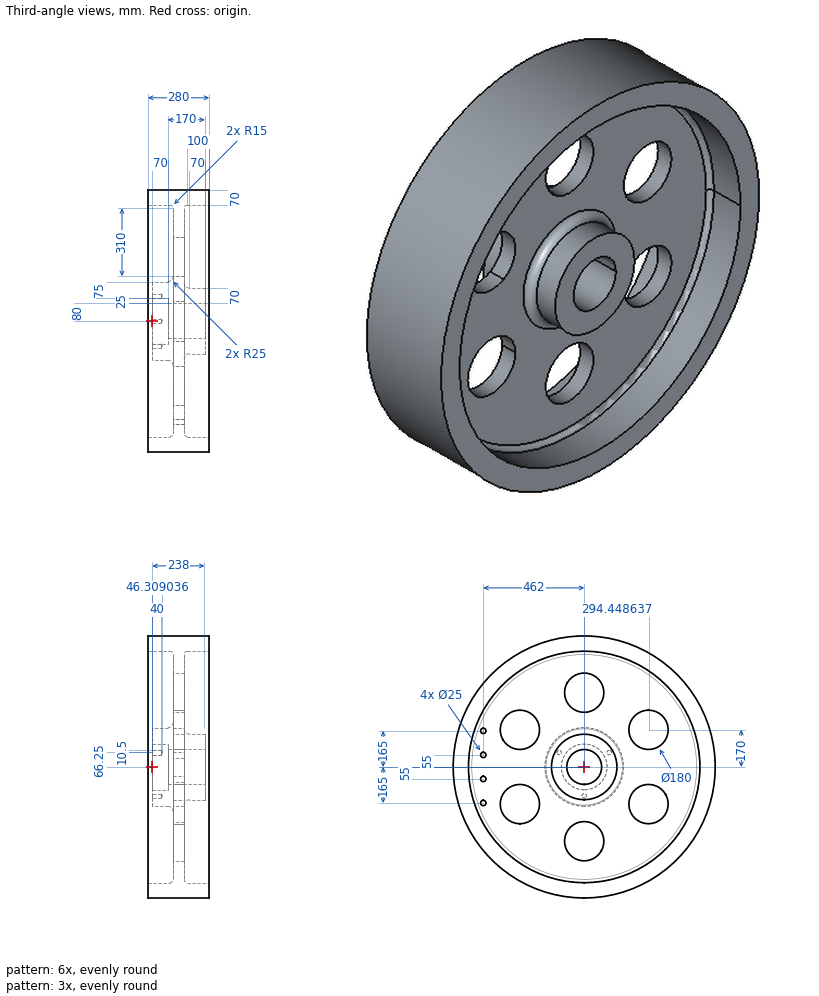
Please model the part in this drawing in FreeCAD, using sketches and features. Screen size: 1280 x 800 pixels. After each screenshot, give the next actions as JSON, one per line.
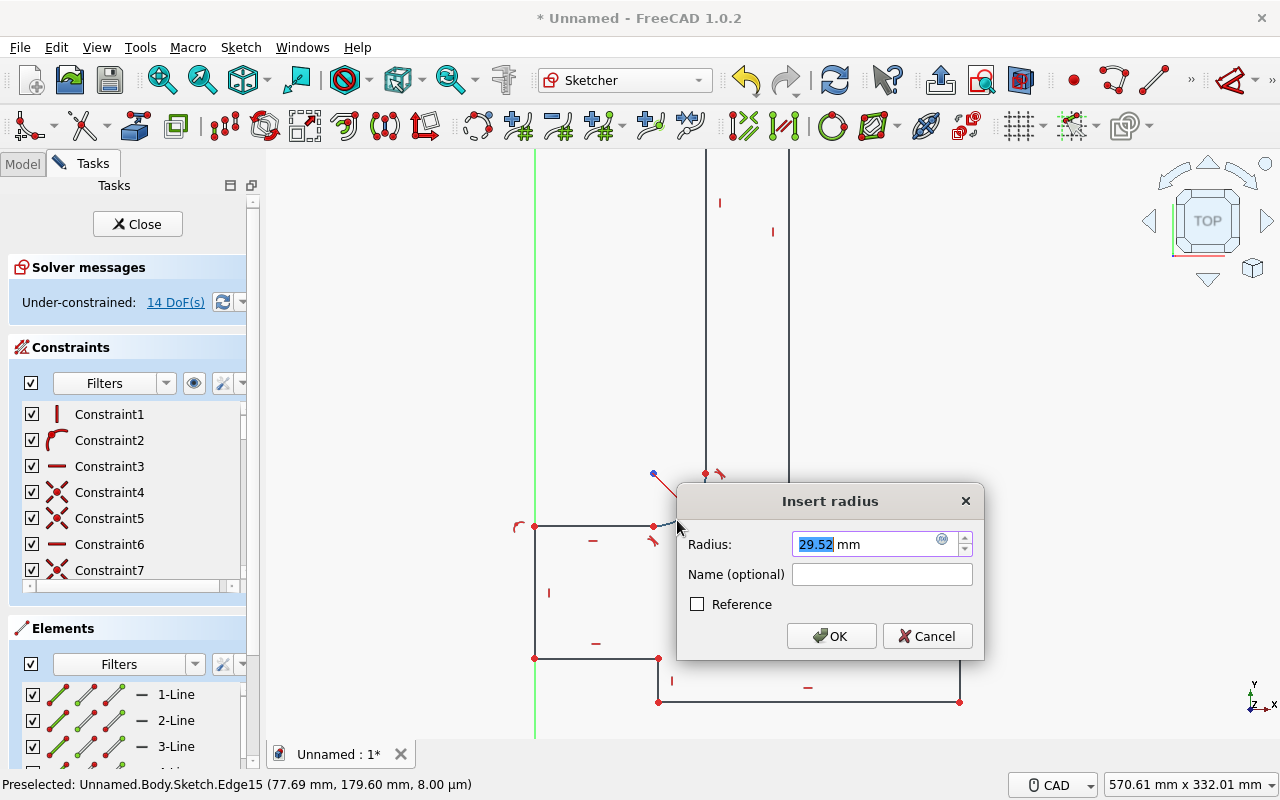
{"action": "type", "text": "25"}
{"action": "key", "text": "Return"}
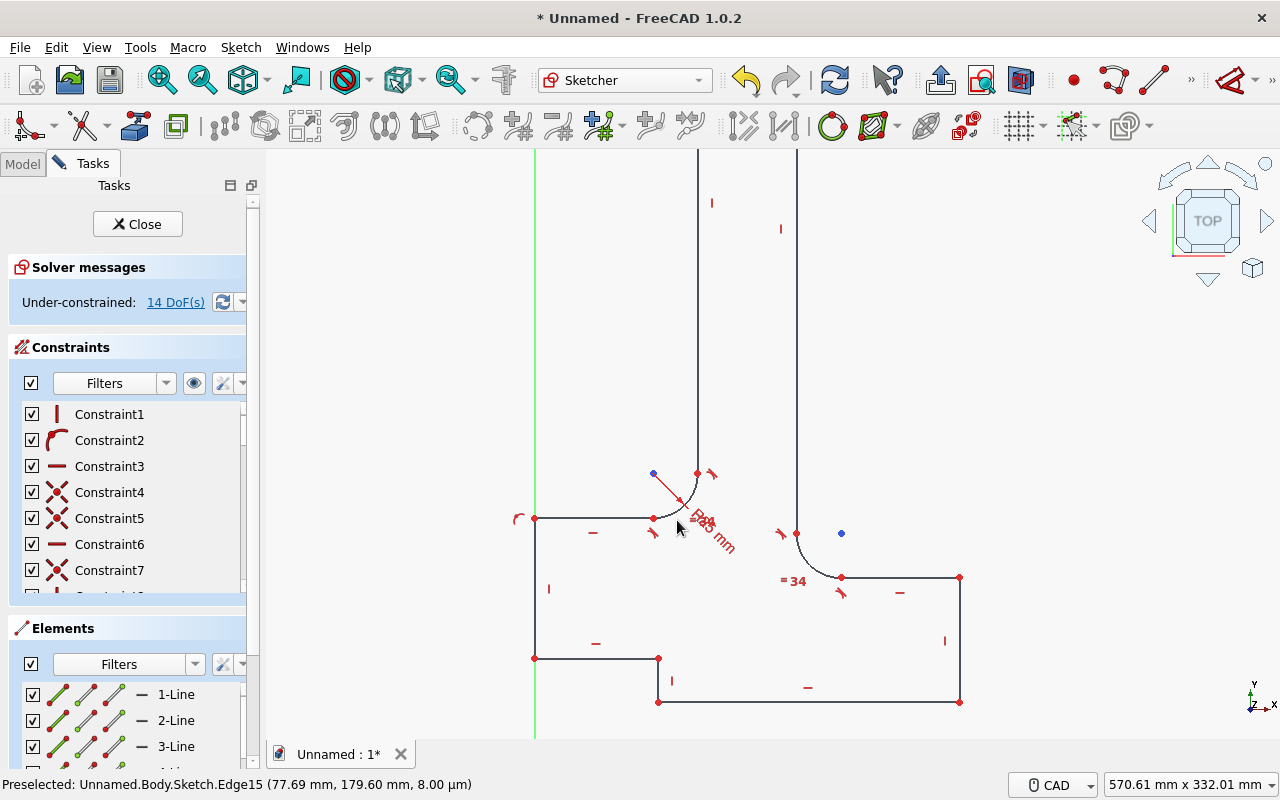
{"action": "scroll", "coordinate": [679, 523], "scroll_direction": "down", "scroll_amount": 5}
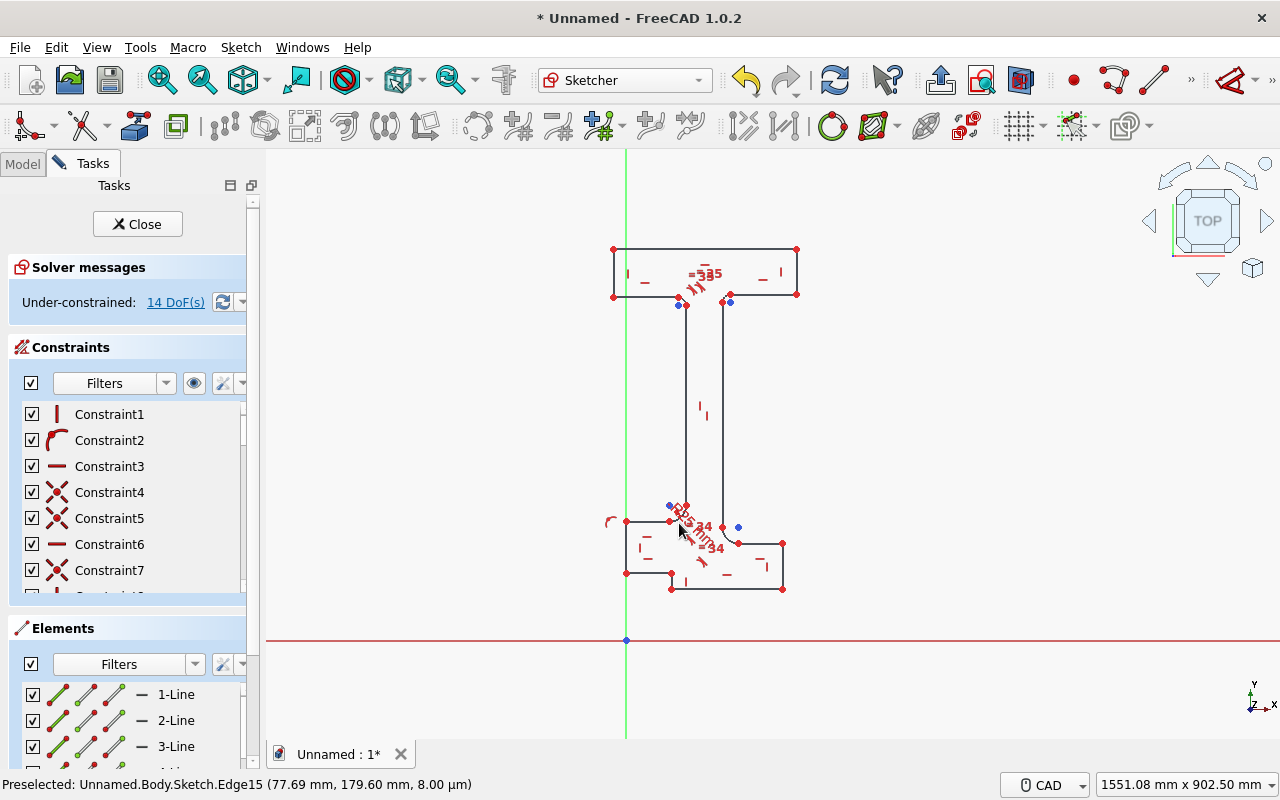
{"action": "scroll", "coordinate": [727, 296], "scroll_direction": "up", "scroll_amount": 7}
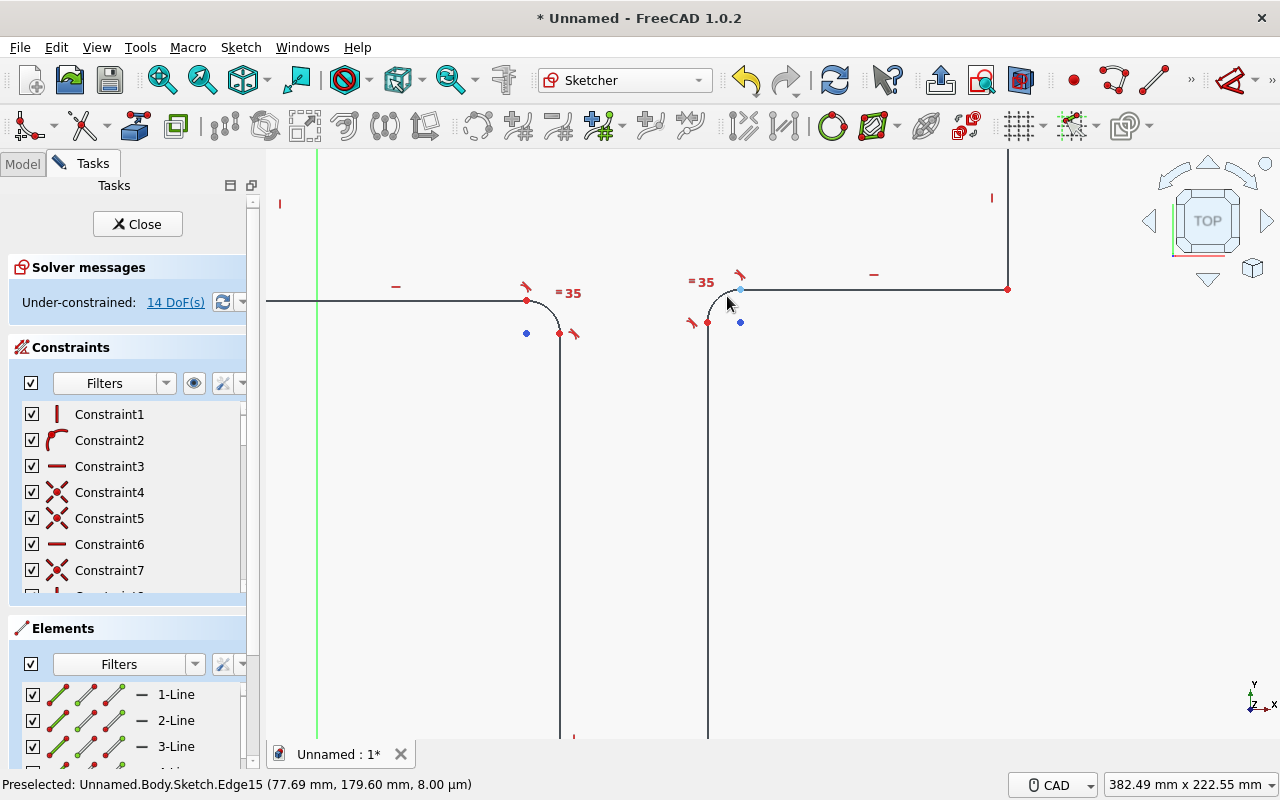
{"action": "left_click", "coordinate": [726, 293]}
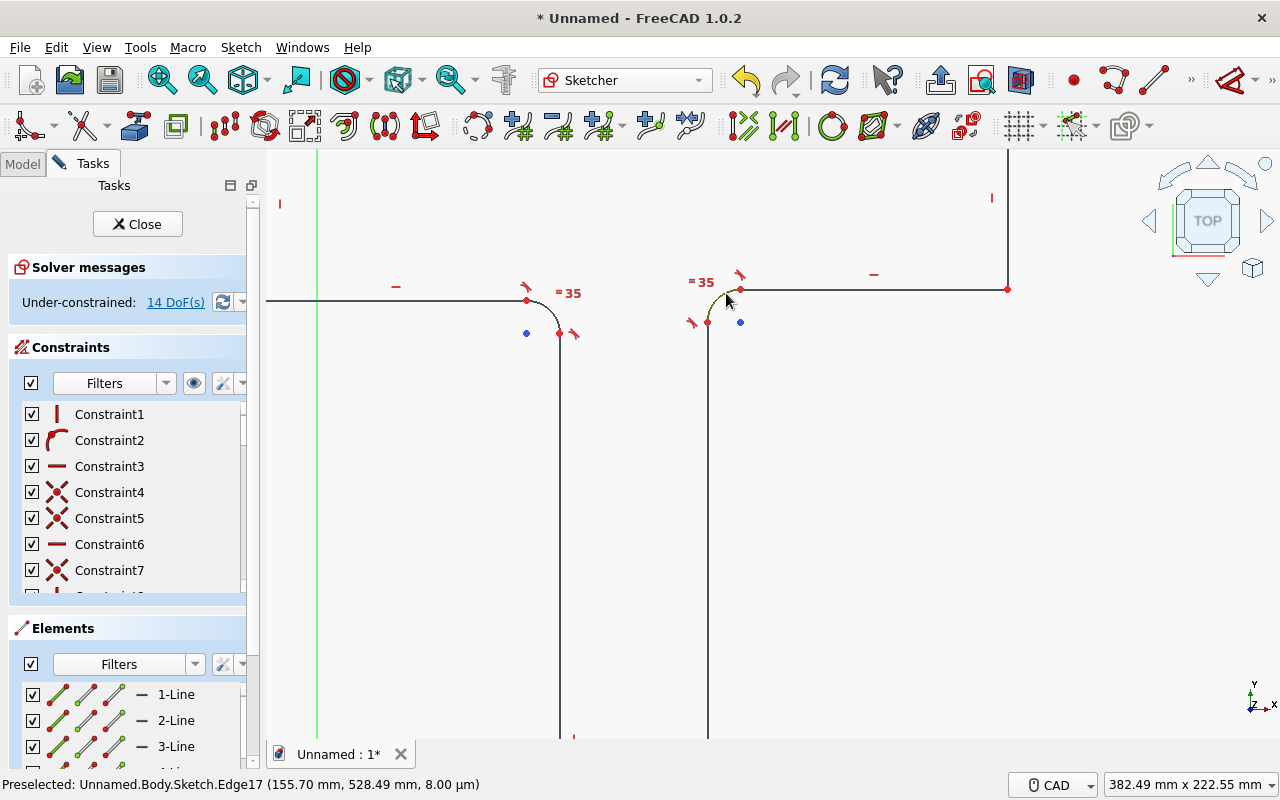
{"action": "left_click", "coordinate": [1258, 80]}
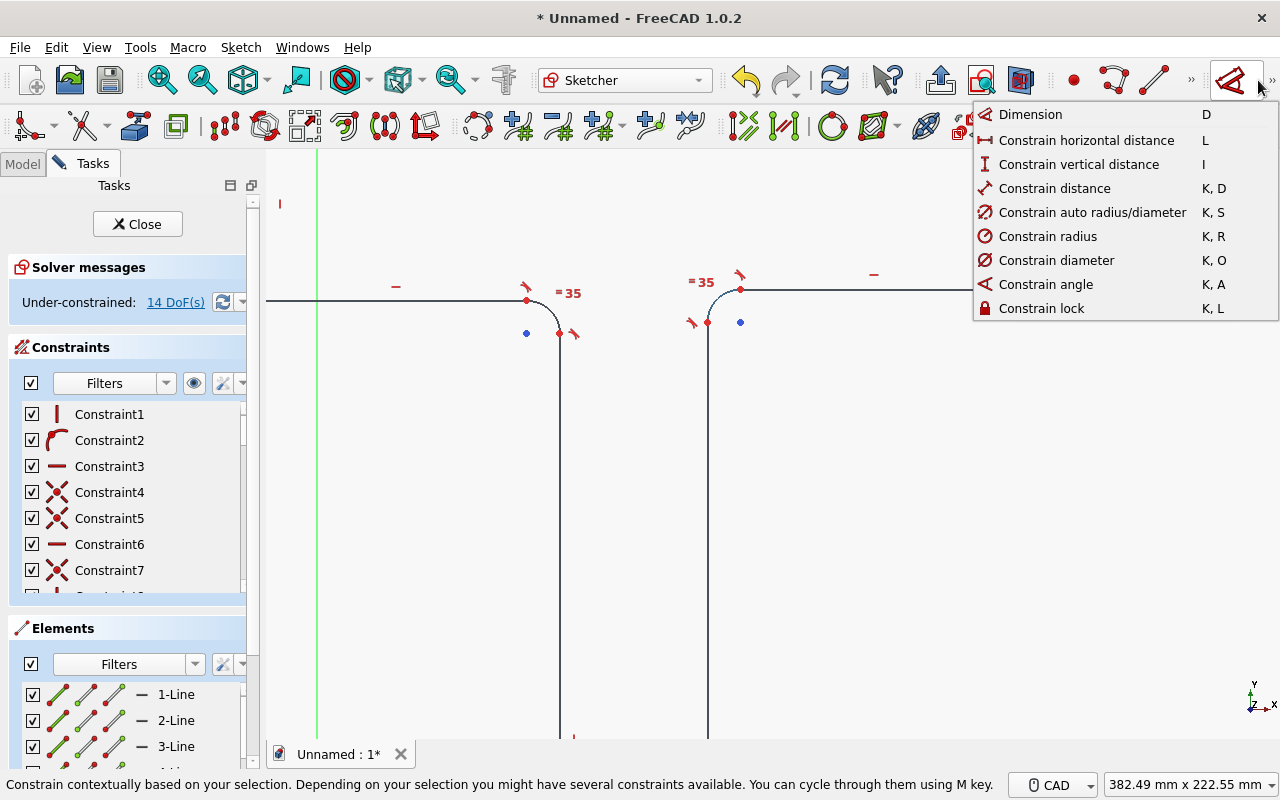
{"action": "left_click", "coordinate": [1126, 236]}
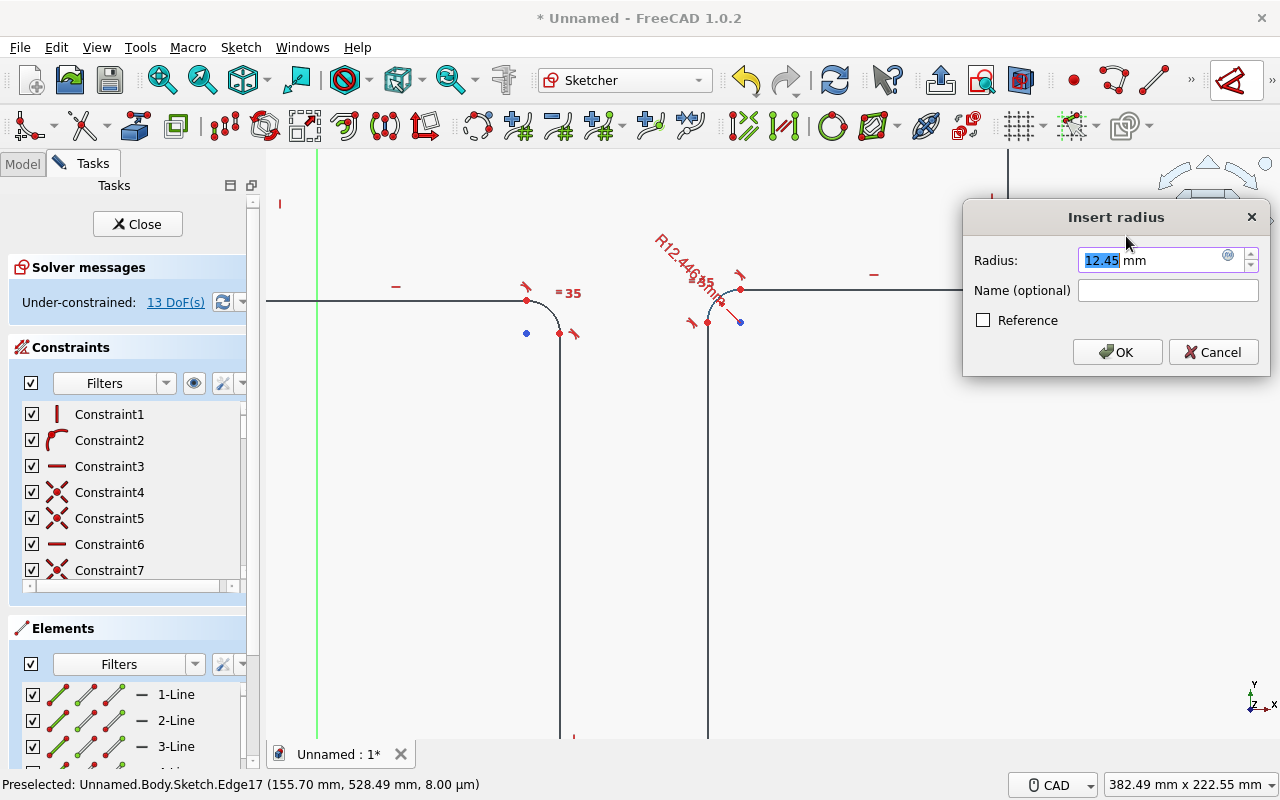
{"action": "type", "text": "15"}
{"action": "key", "text": "Return"}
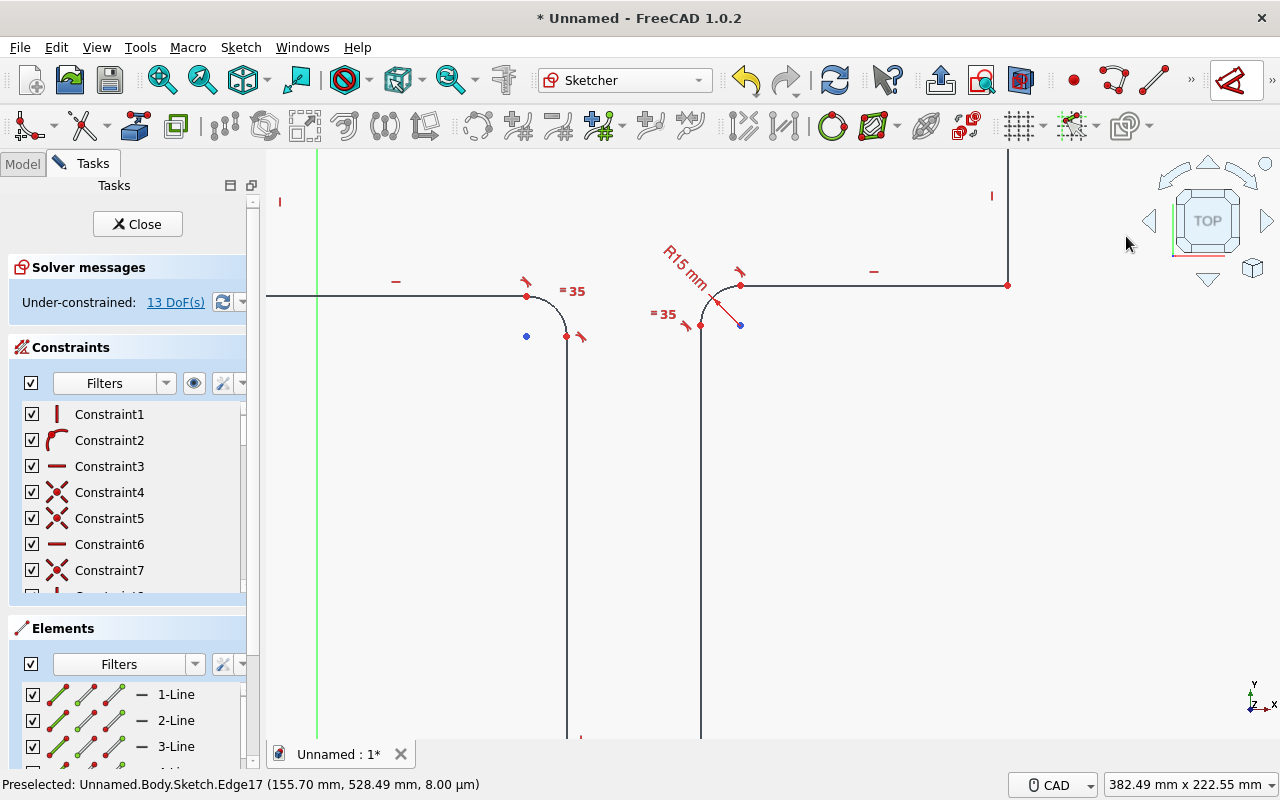
{"action": "scroll", "coordinate": [727, 296], "scroll_direction": "down", "scroll_amount": 7}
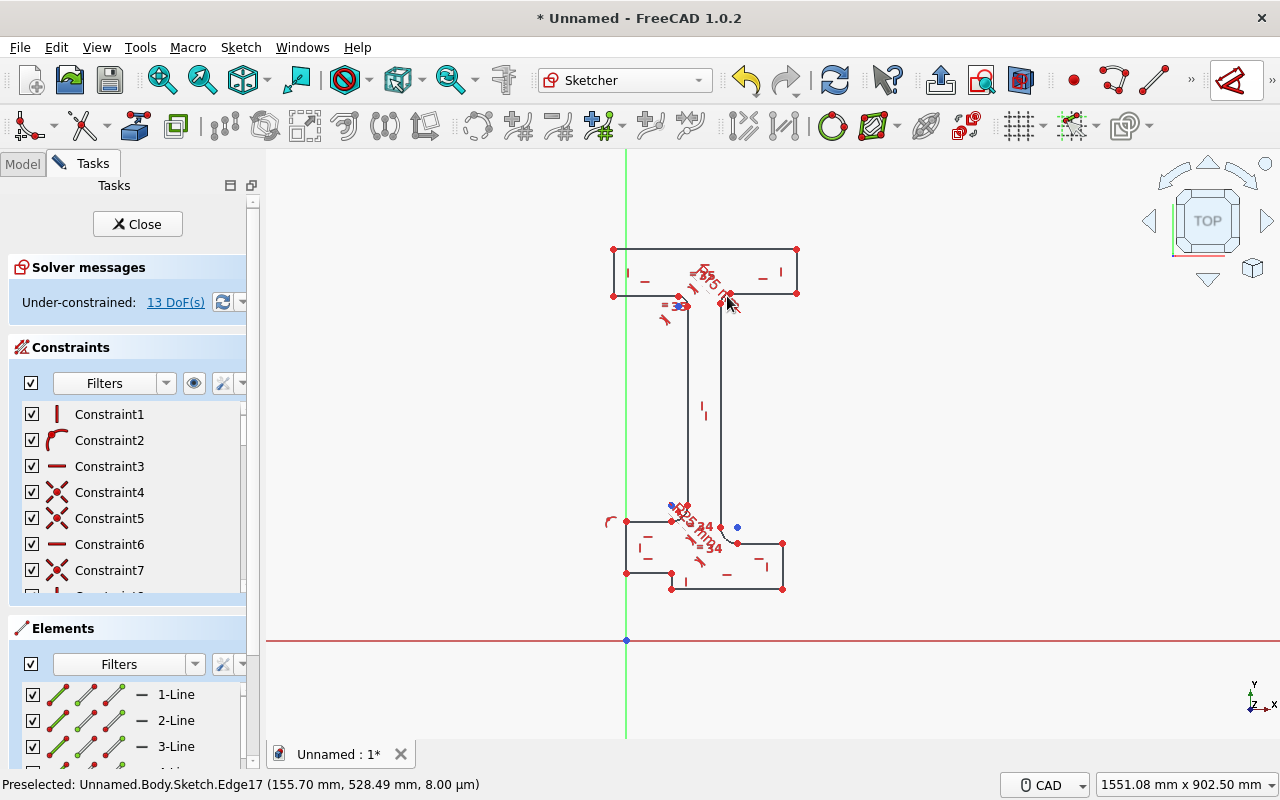
{"action": "left_click", "coordinate": [658, 522]}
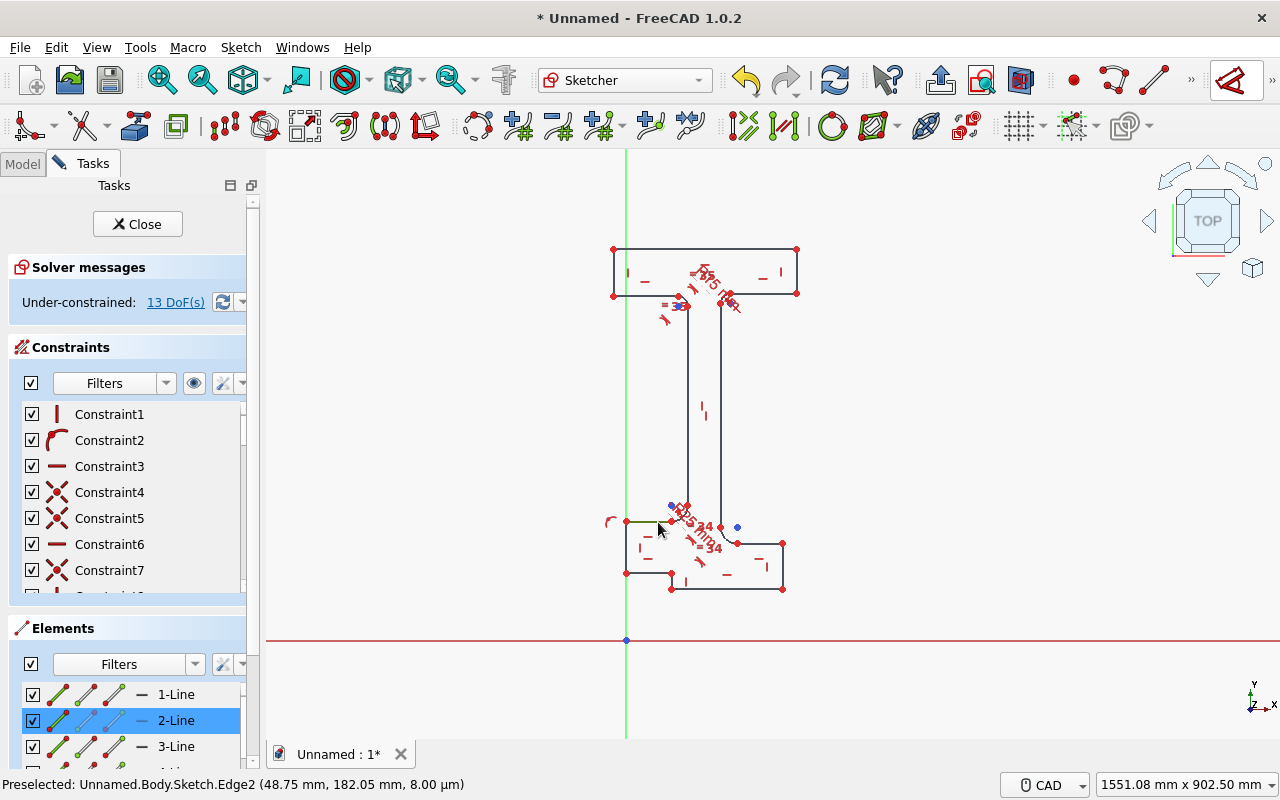
{"action": "left_click", "coordinate": [1258, 80]}